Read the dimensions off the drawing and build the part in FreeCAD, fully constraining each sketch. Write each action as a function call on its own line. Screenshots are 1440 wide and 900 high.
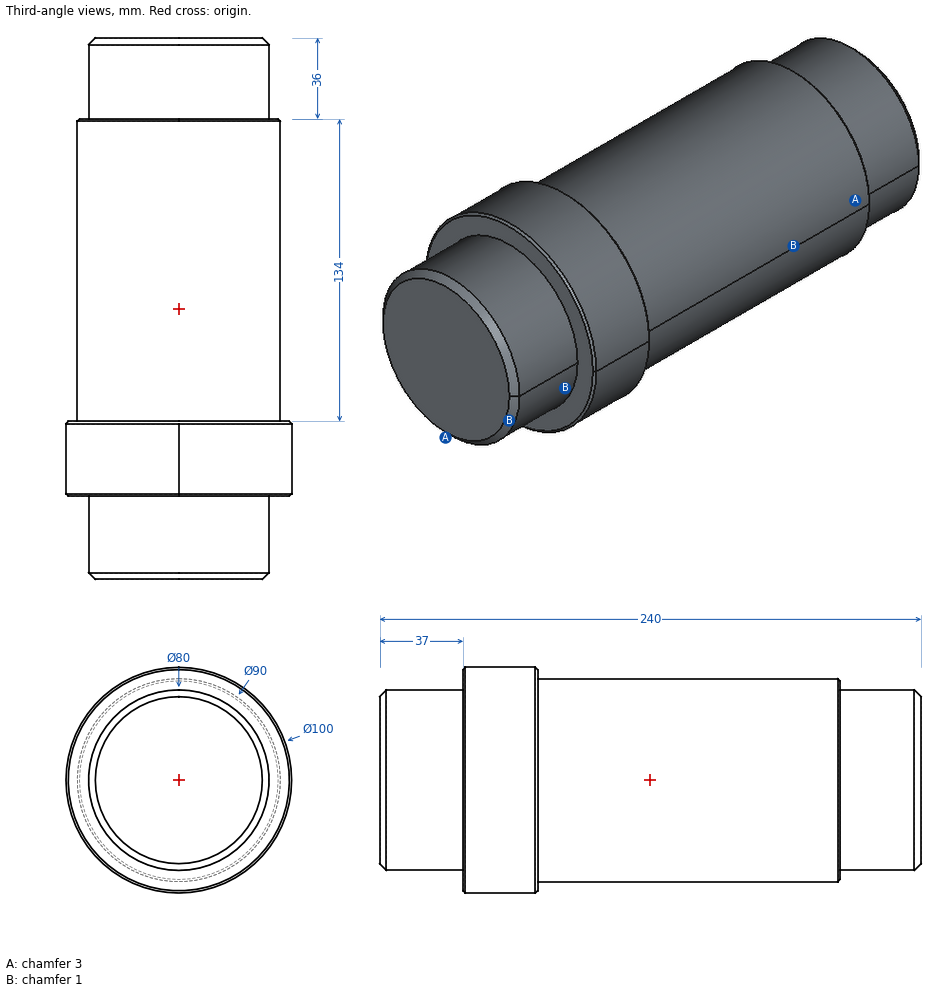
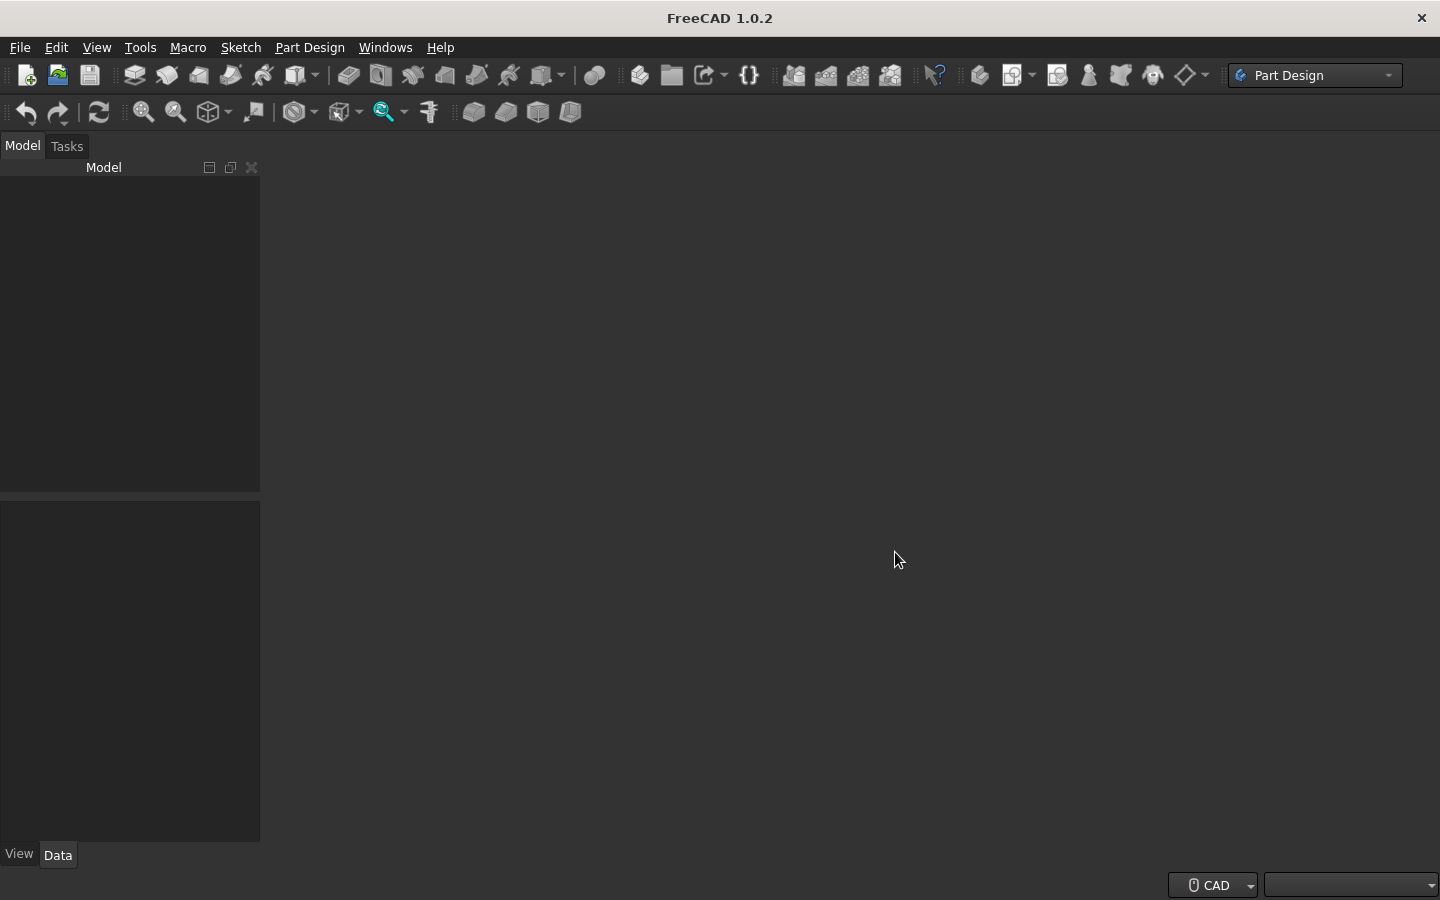
click(26, 76)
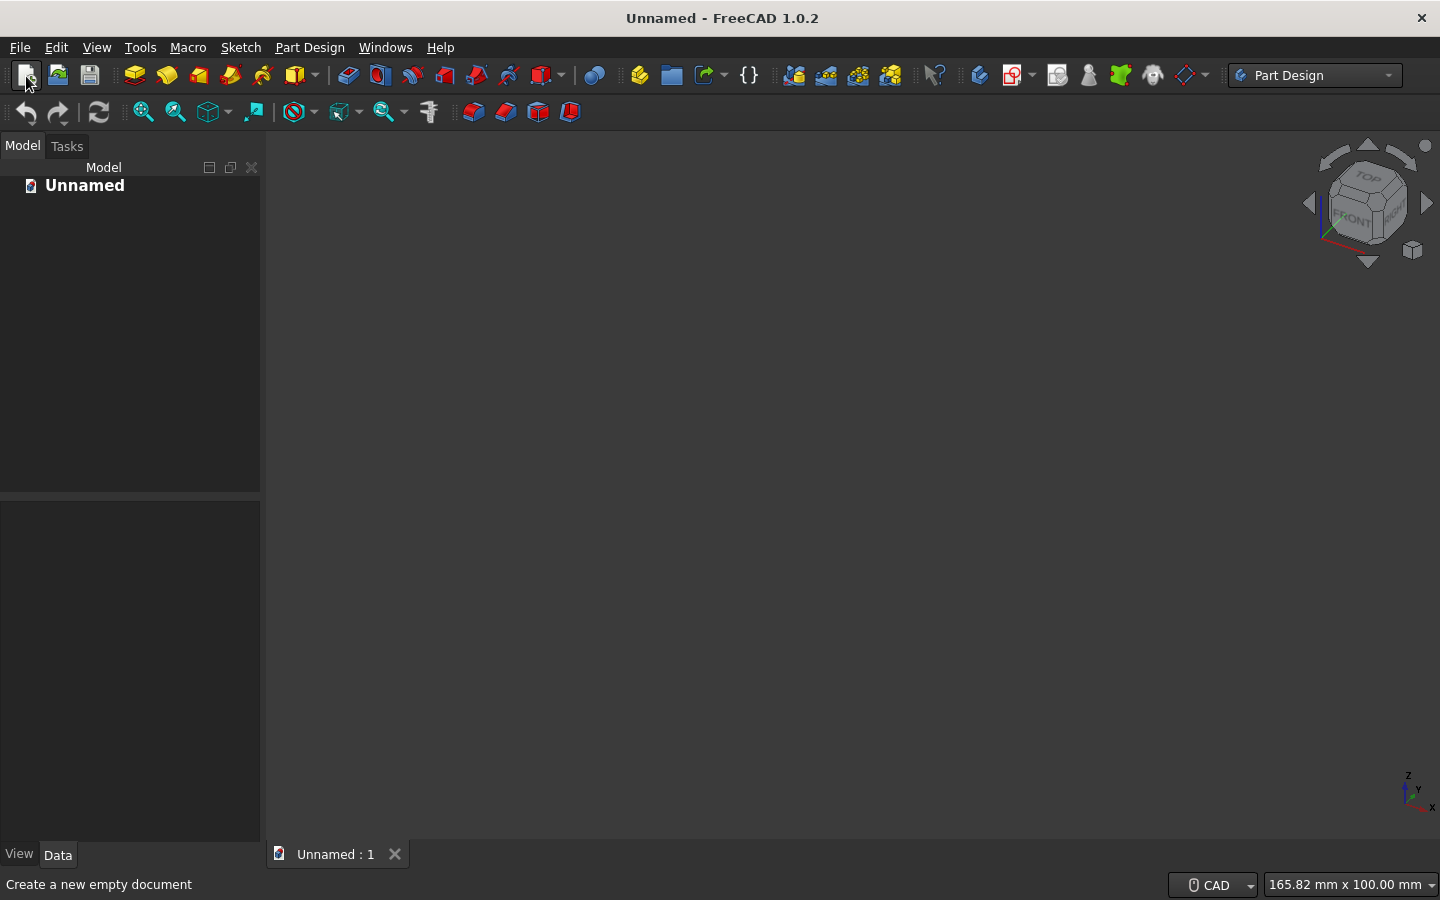
click(1012, 76)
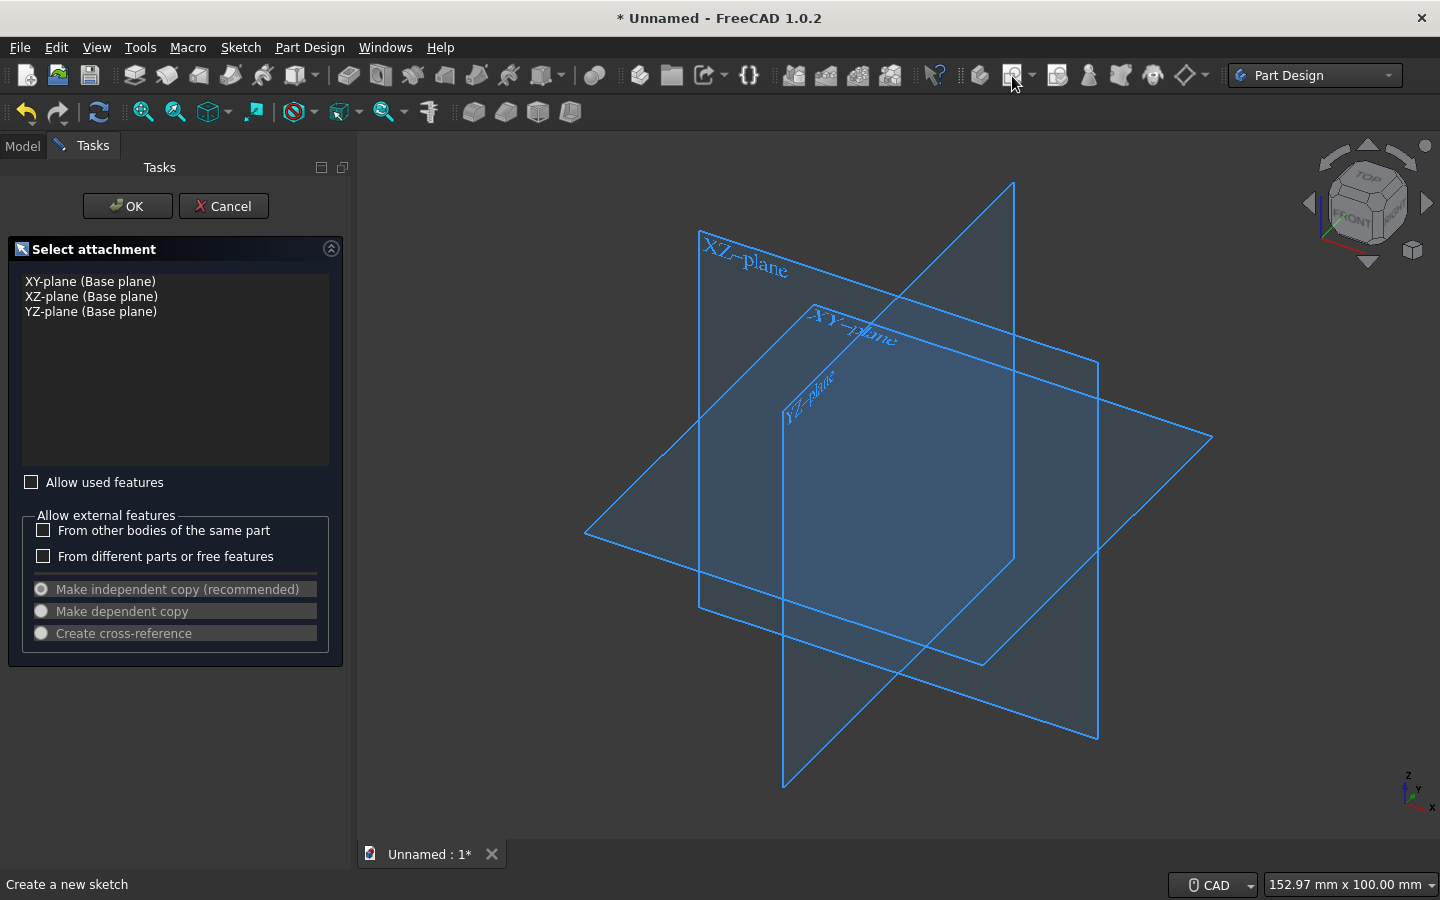
click(82, 296)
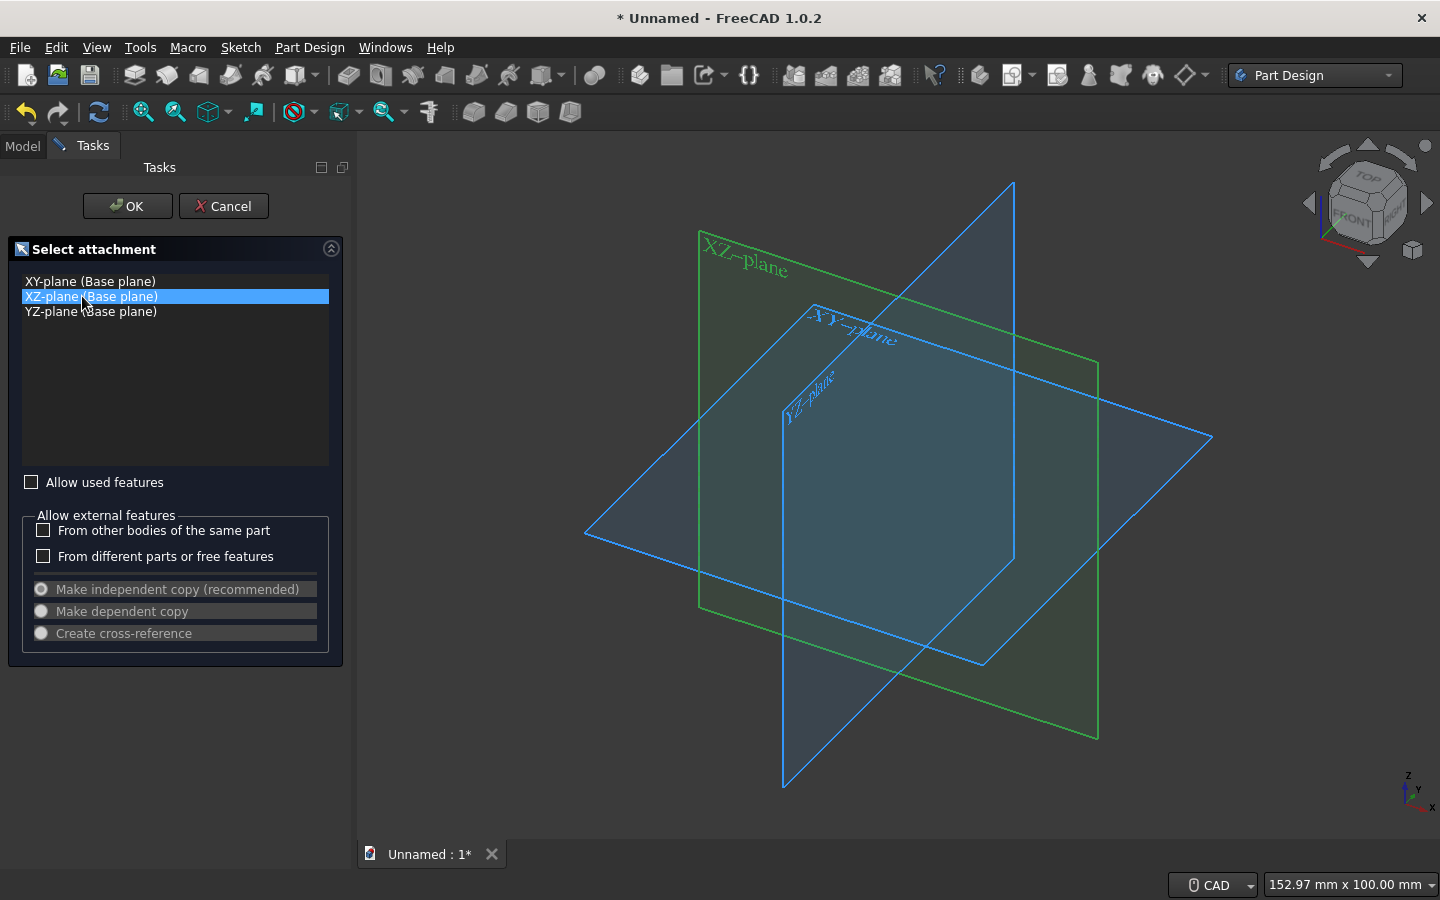
click(128, 206)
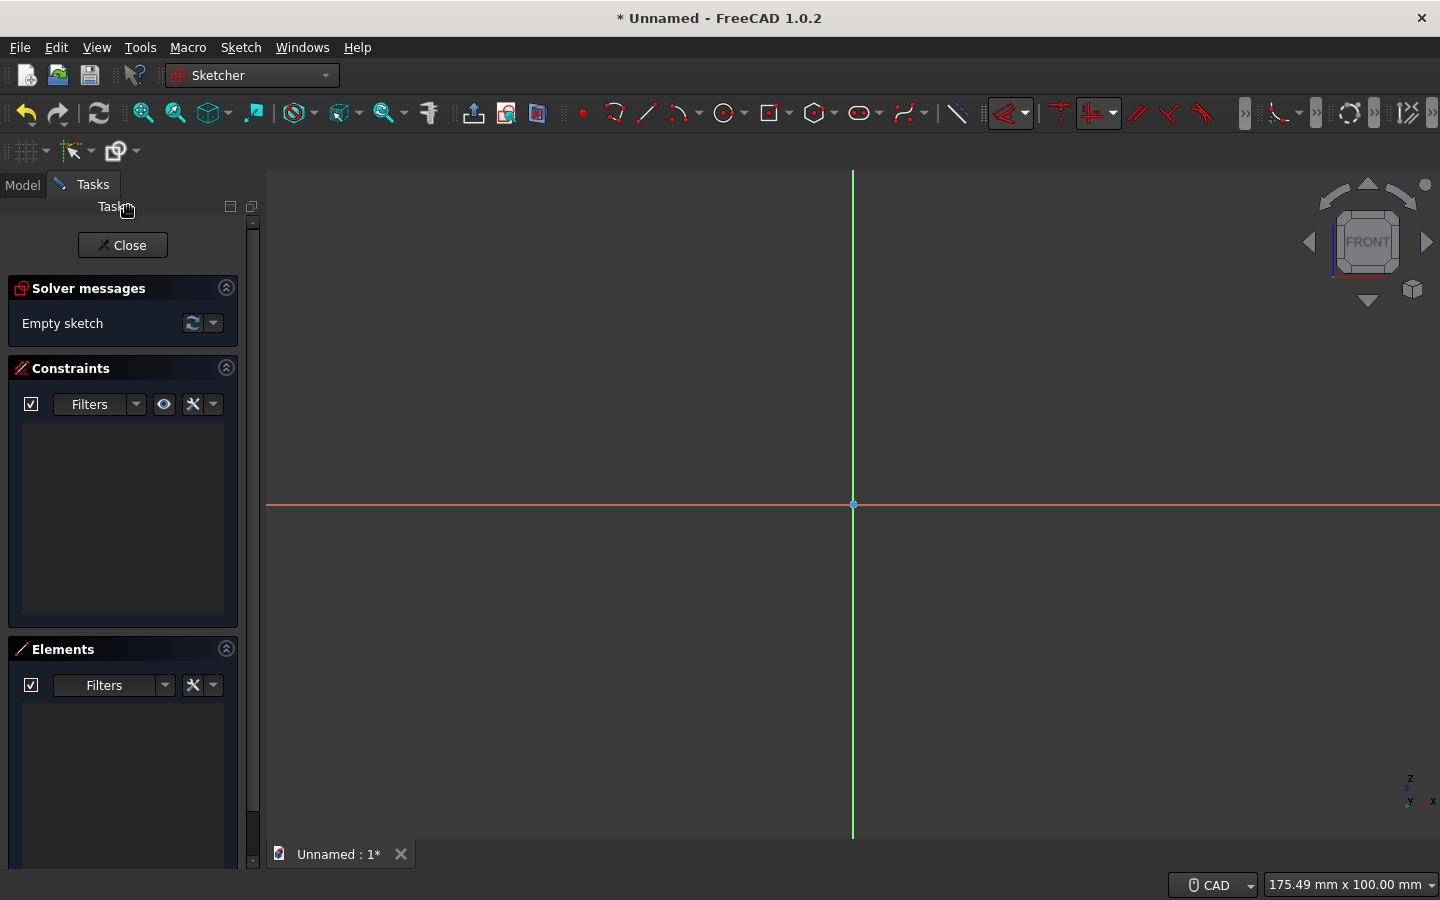
scroll(645, 504, down, 2)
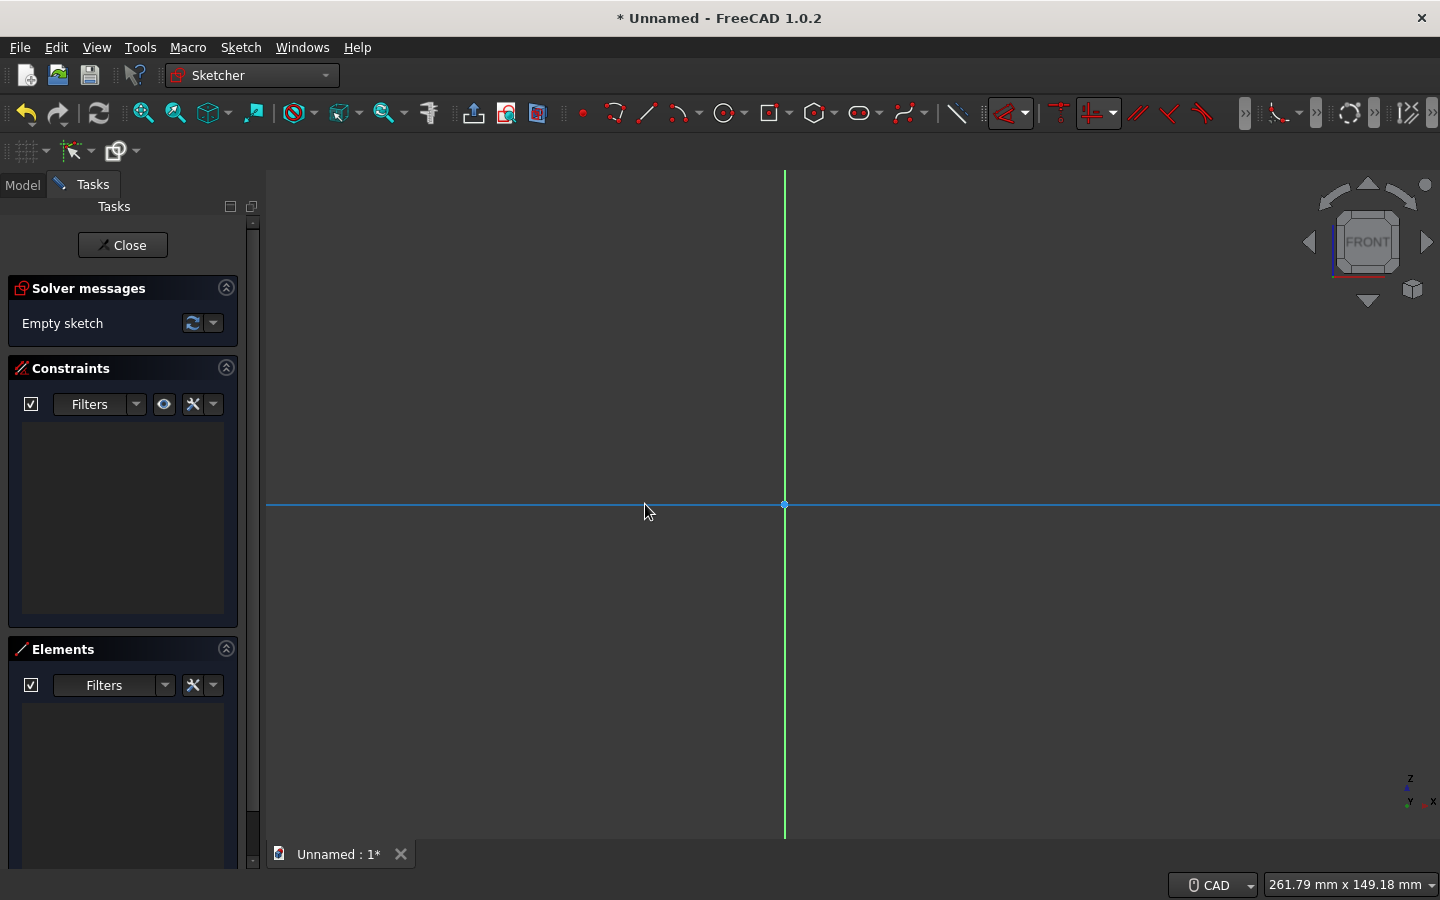
click(724, 114)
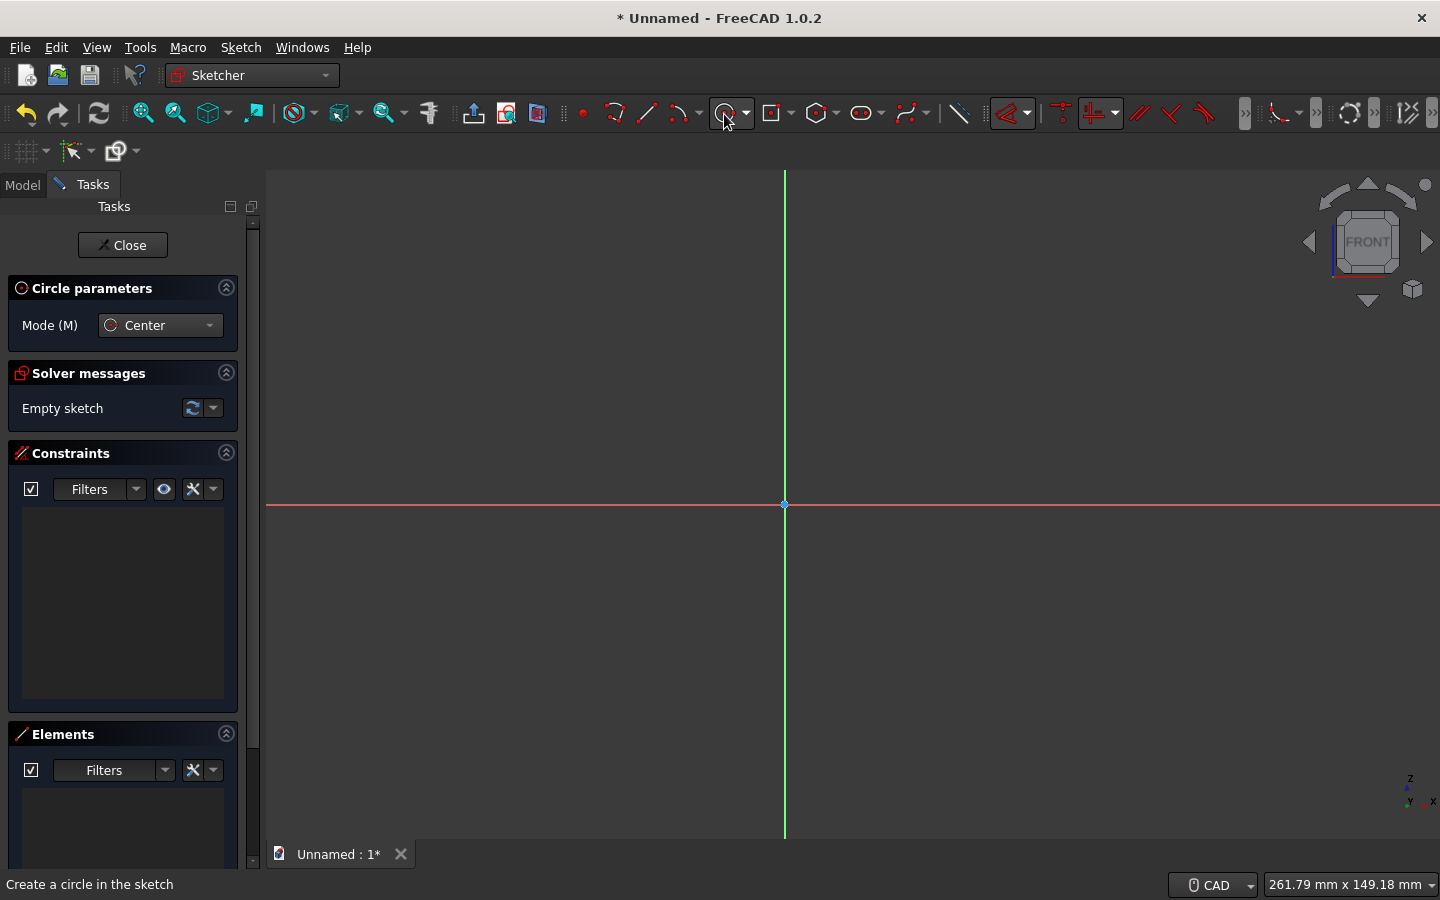
click(785, 504)
click(943, 346)
key(Escape)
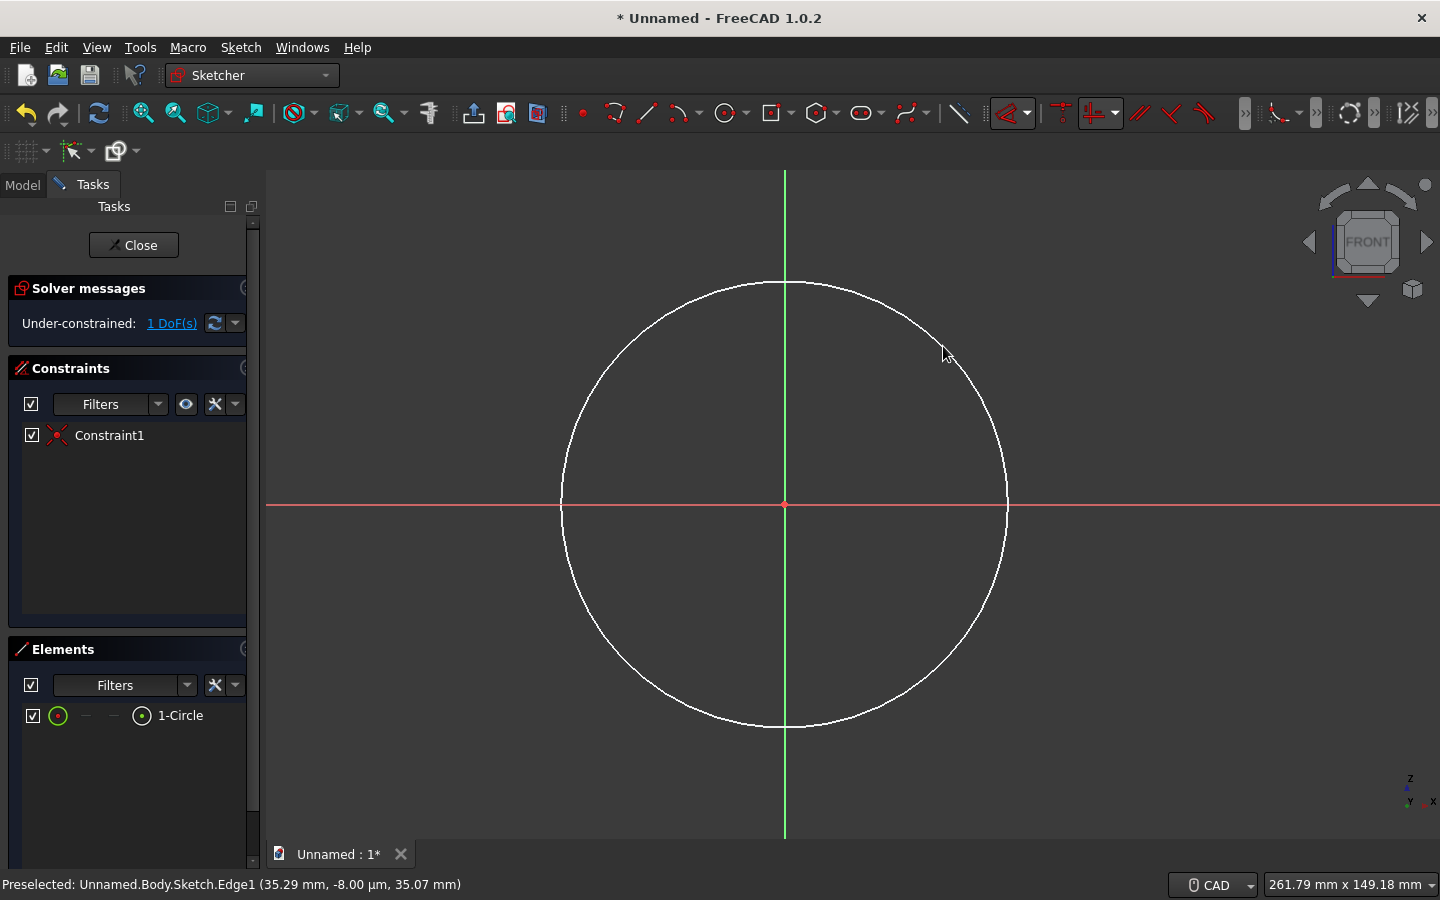
key(d)